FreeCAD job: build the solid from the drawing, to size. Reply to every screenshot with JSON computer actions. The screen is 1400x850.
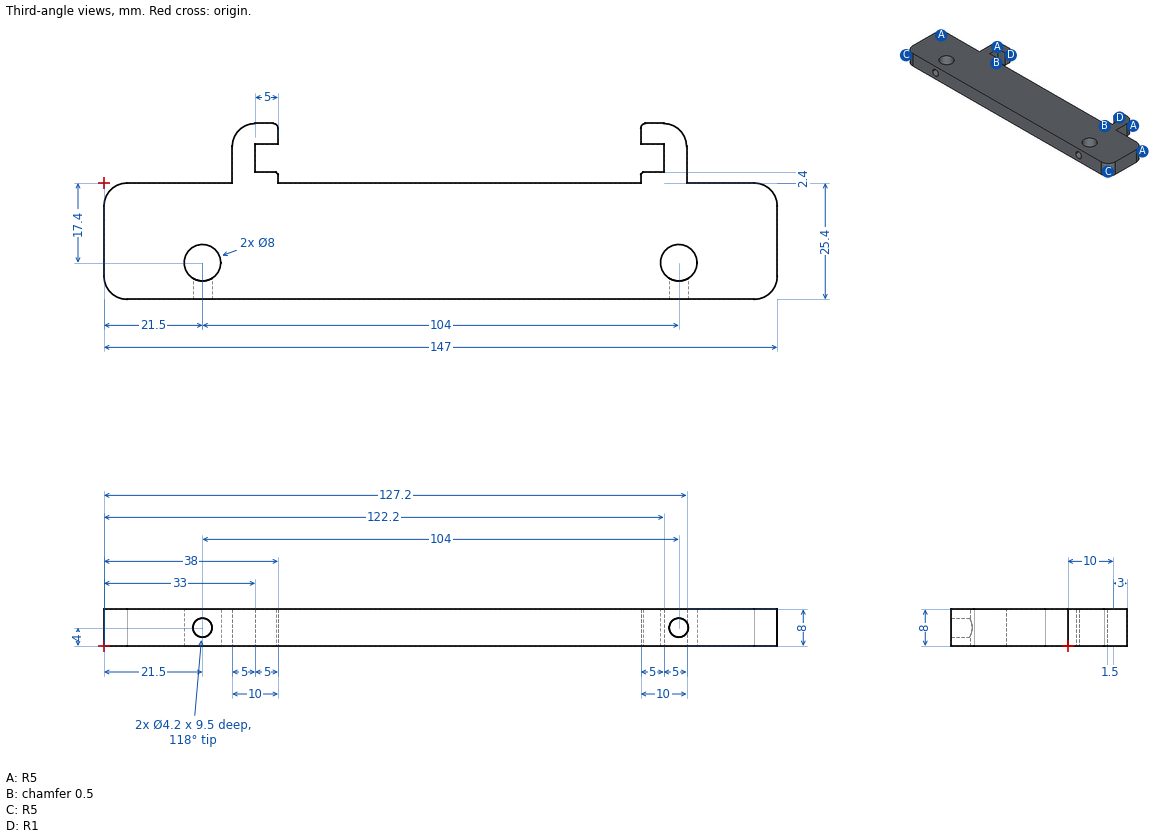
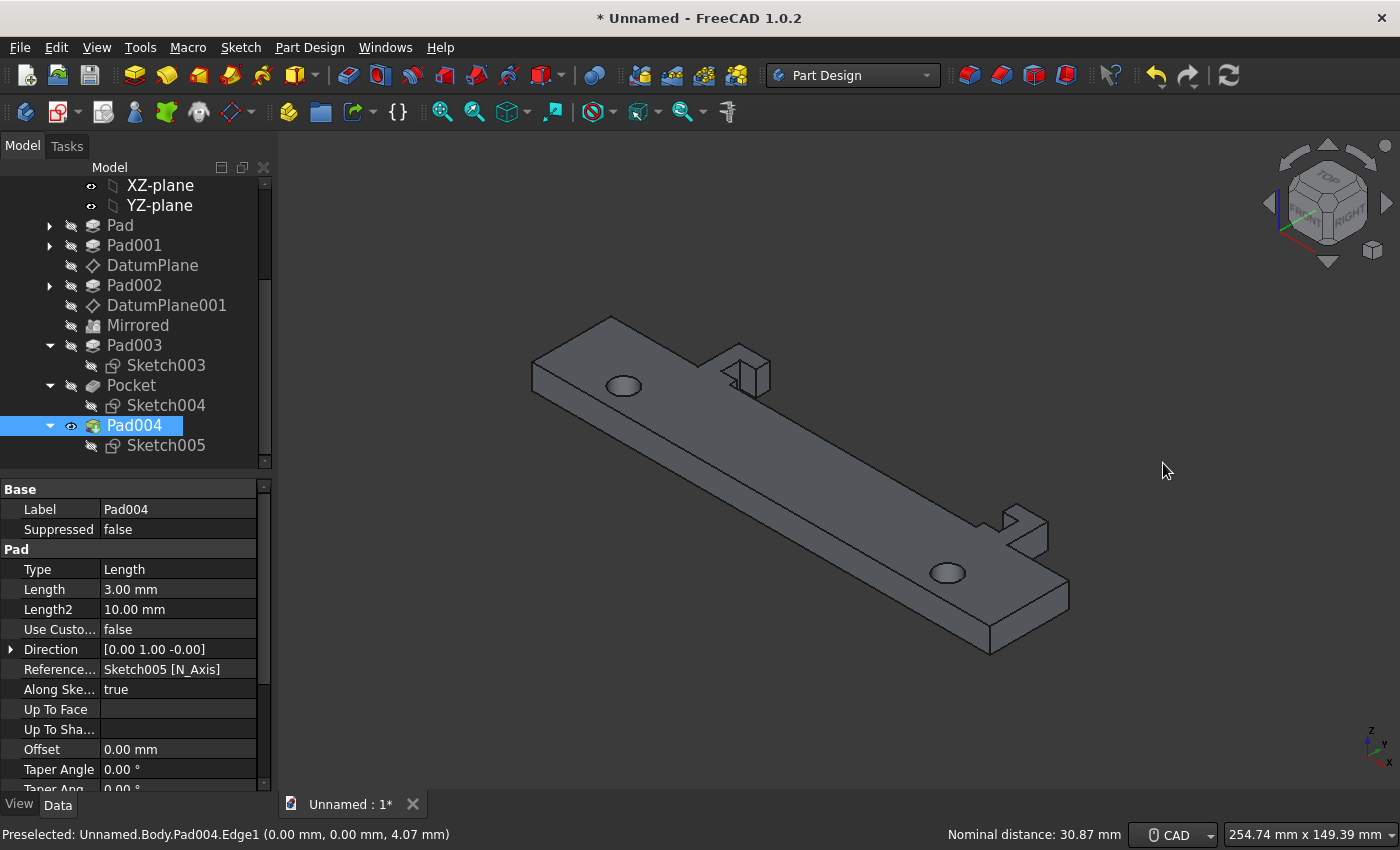
{"action": "key", "text": "2"}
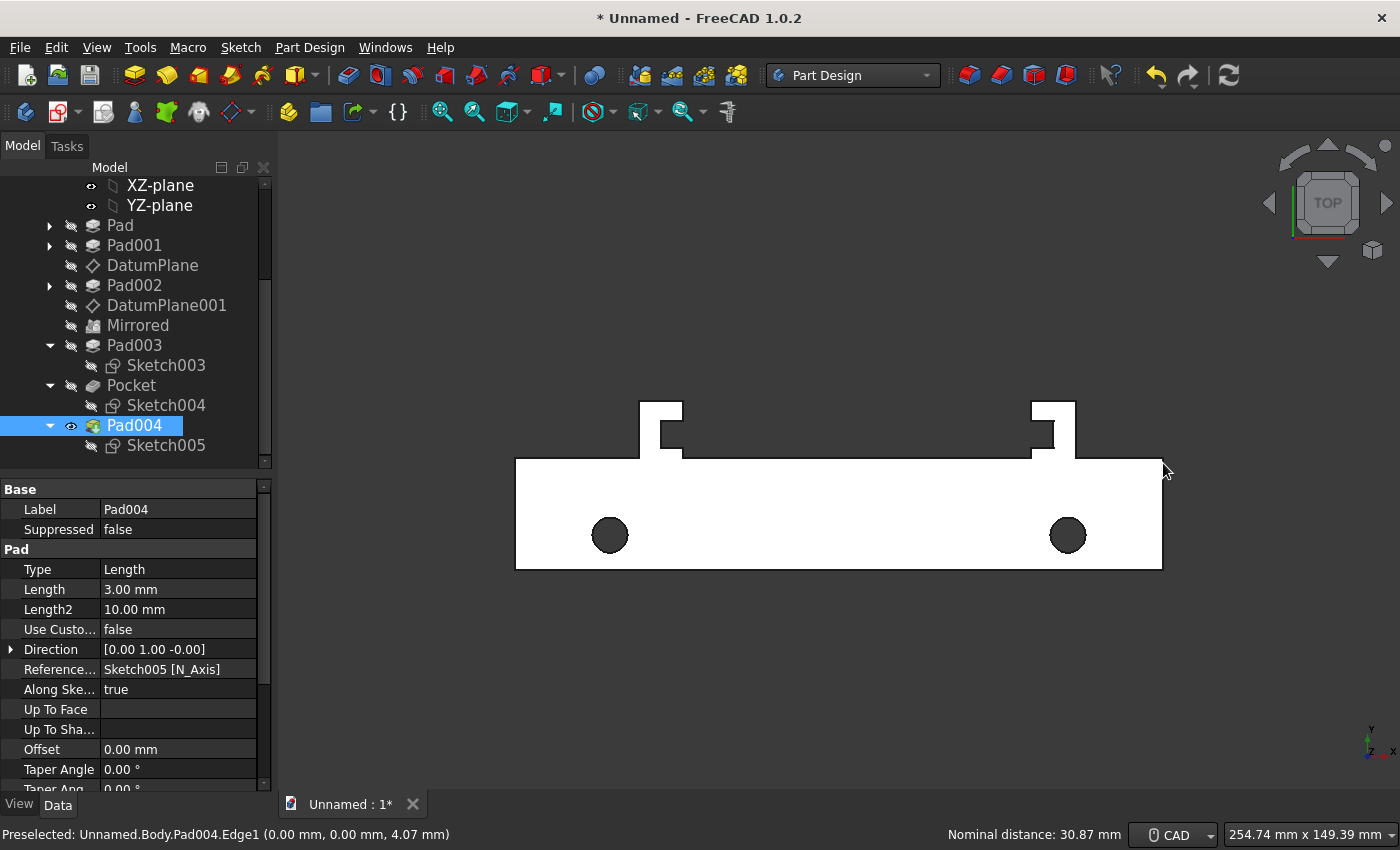
{"action": "key", "text": "1"}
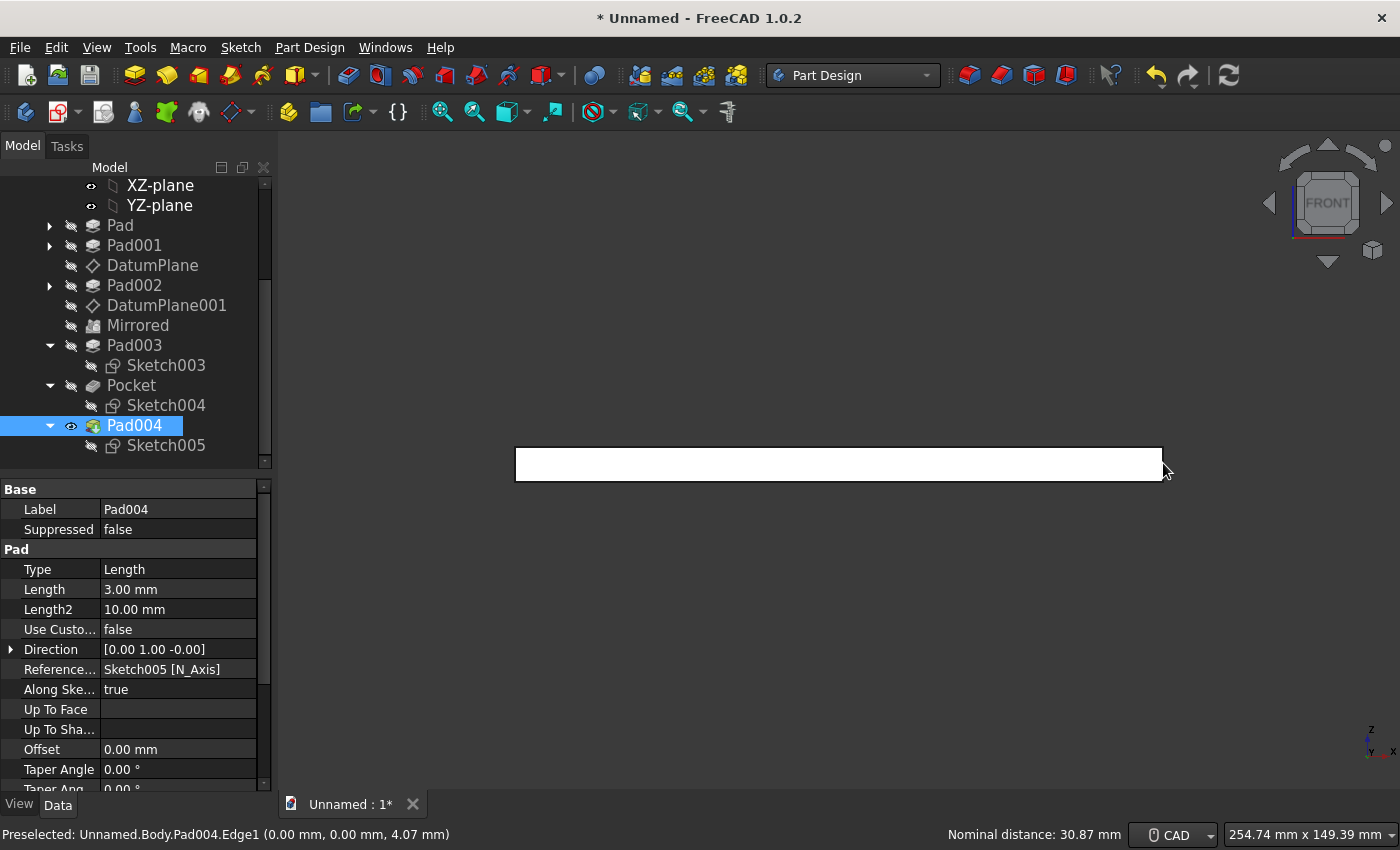
{"action": "key", "text": "3"}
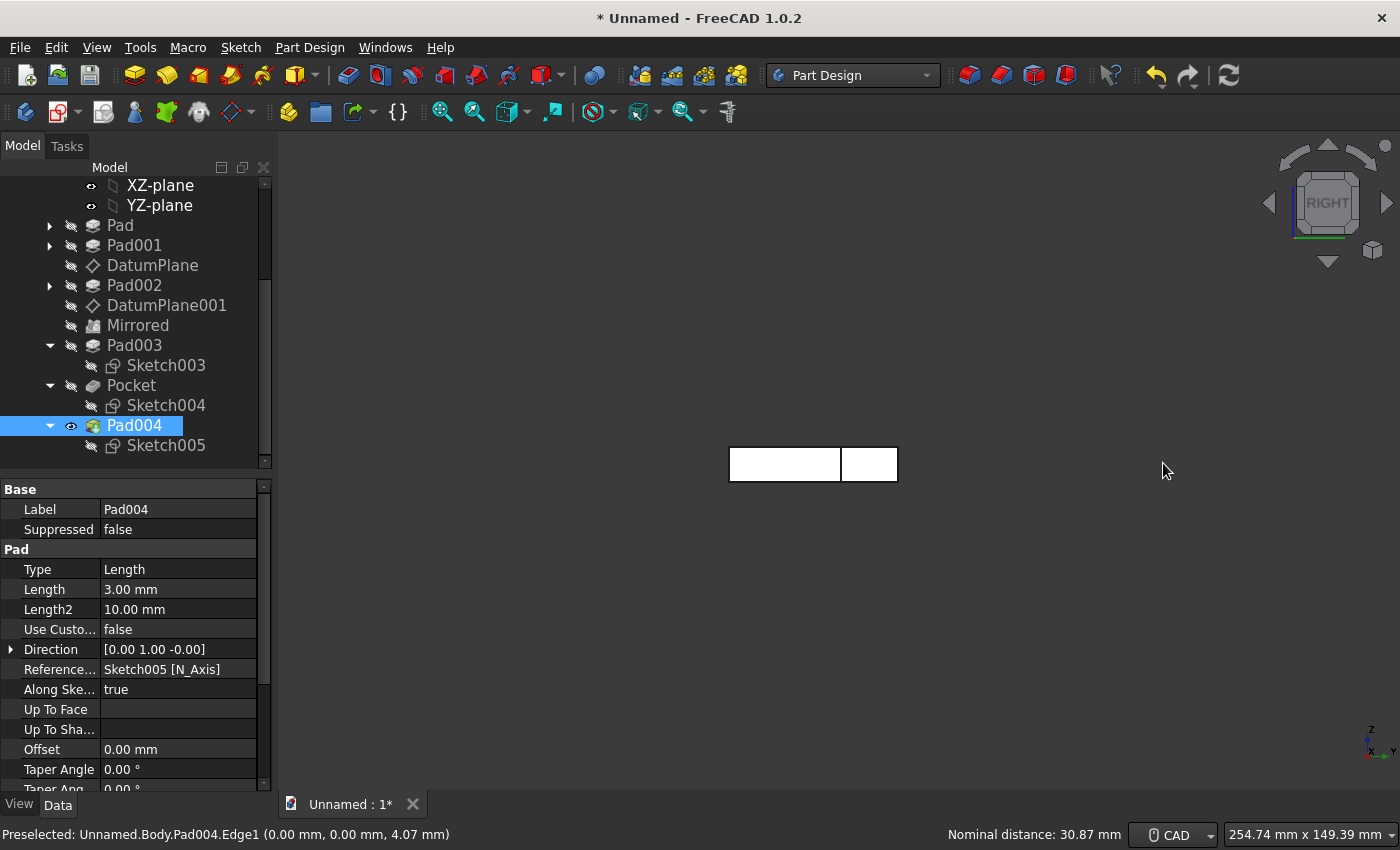
{"action": "left_click", "coordinate": [444, 112]}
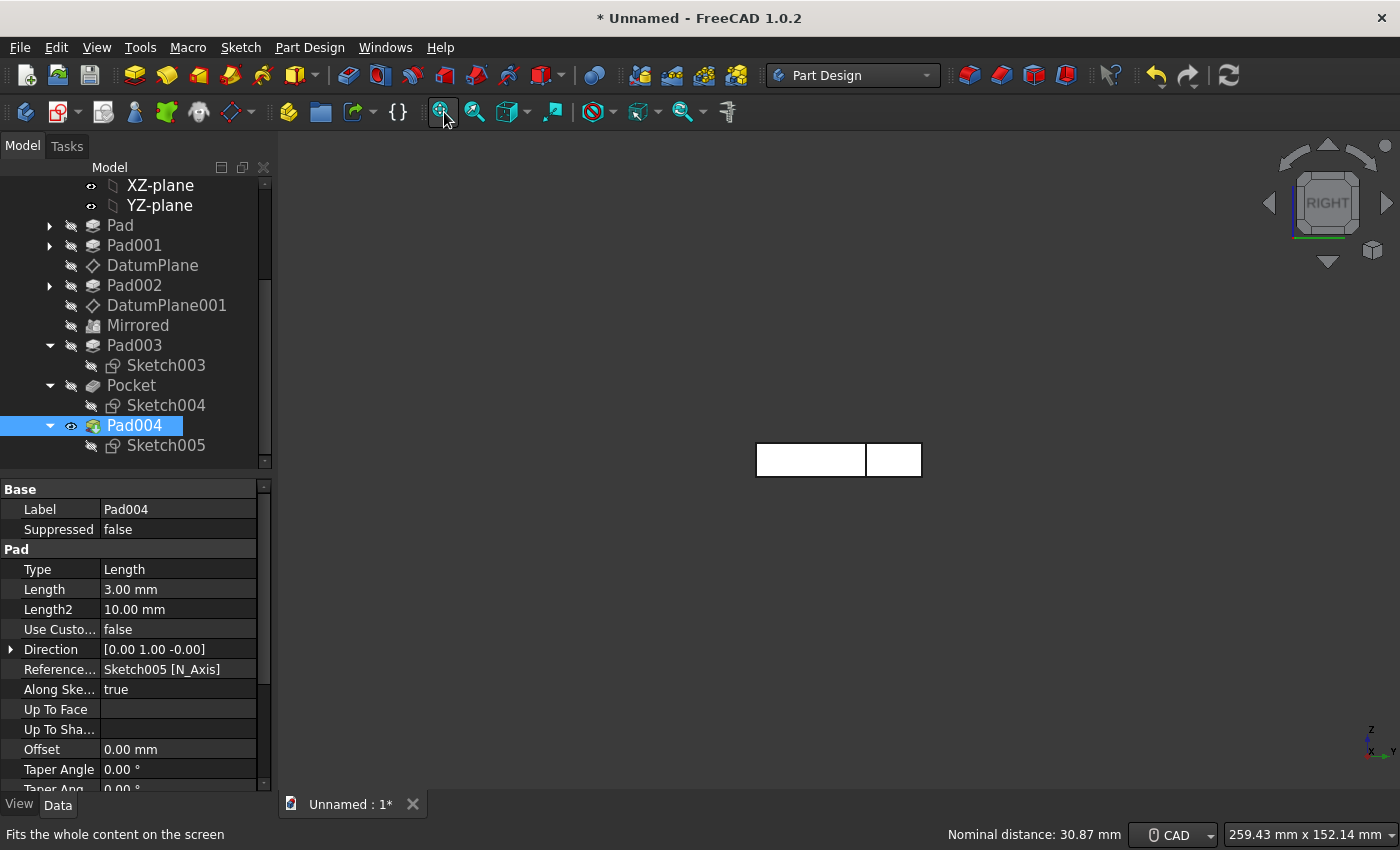
{"action": "left_click", "coordinate": [922, 459], "text": "ctrl"}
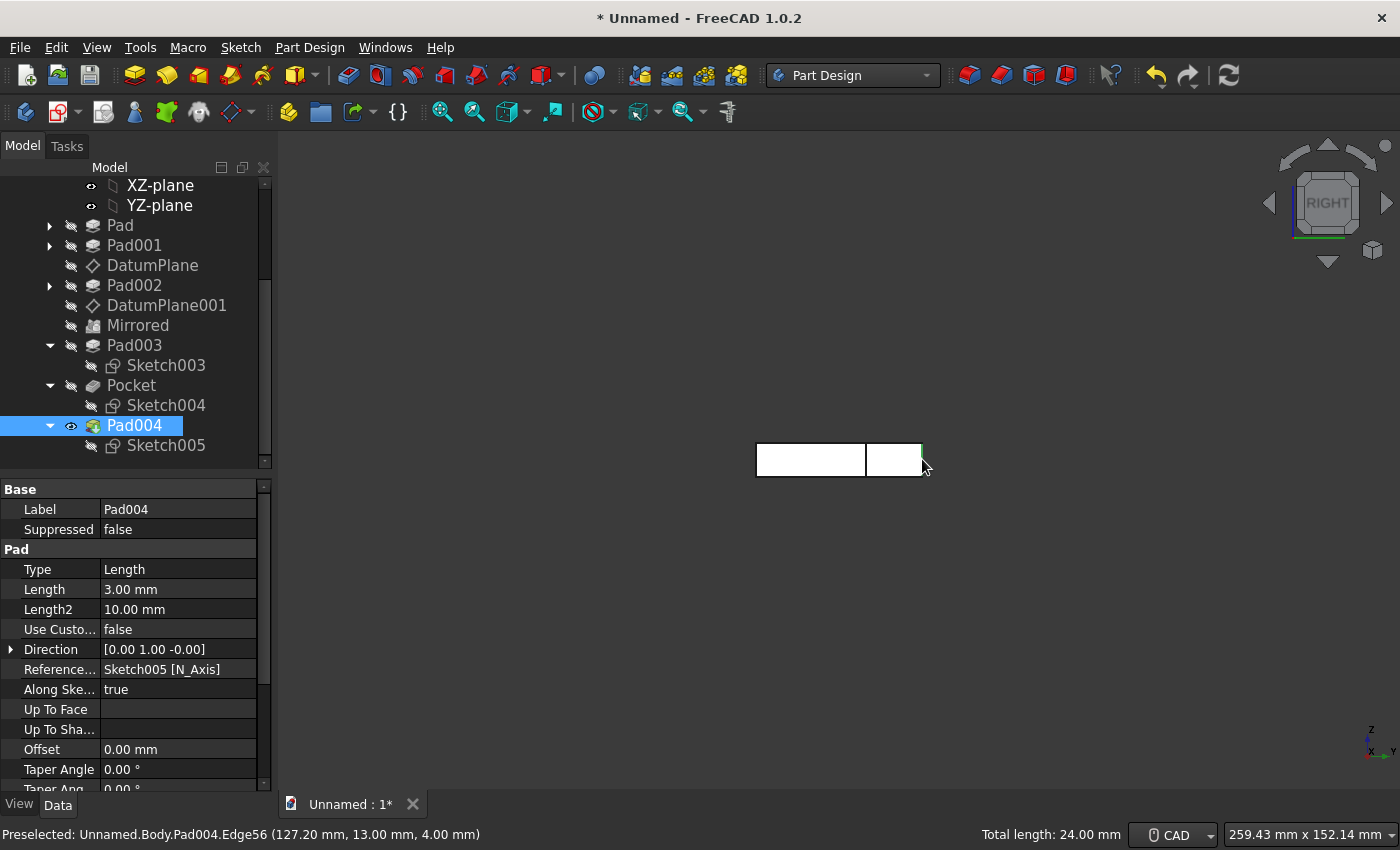
{"action": "left_click", "coordinate": [866, 459], "text": "ctrl"}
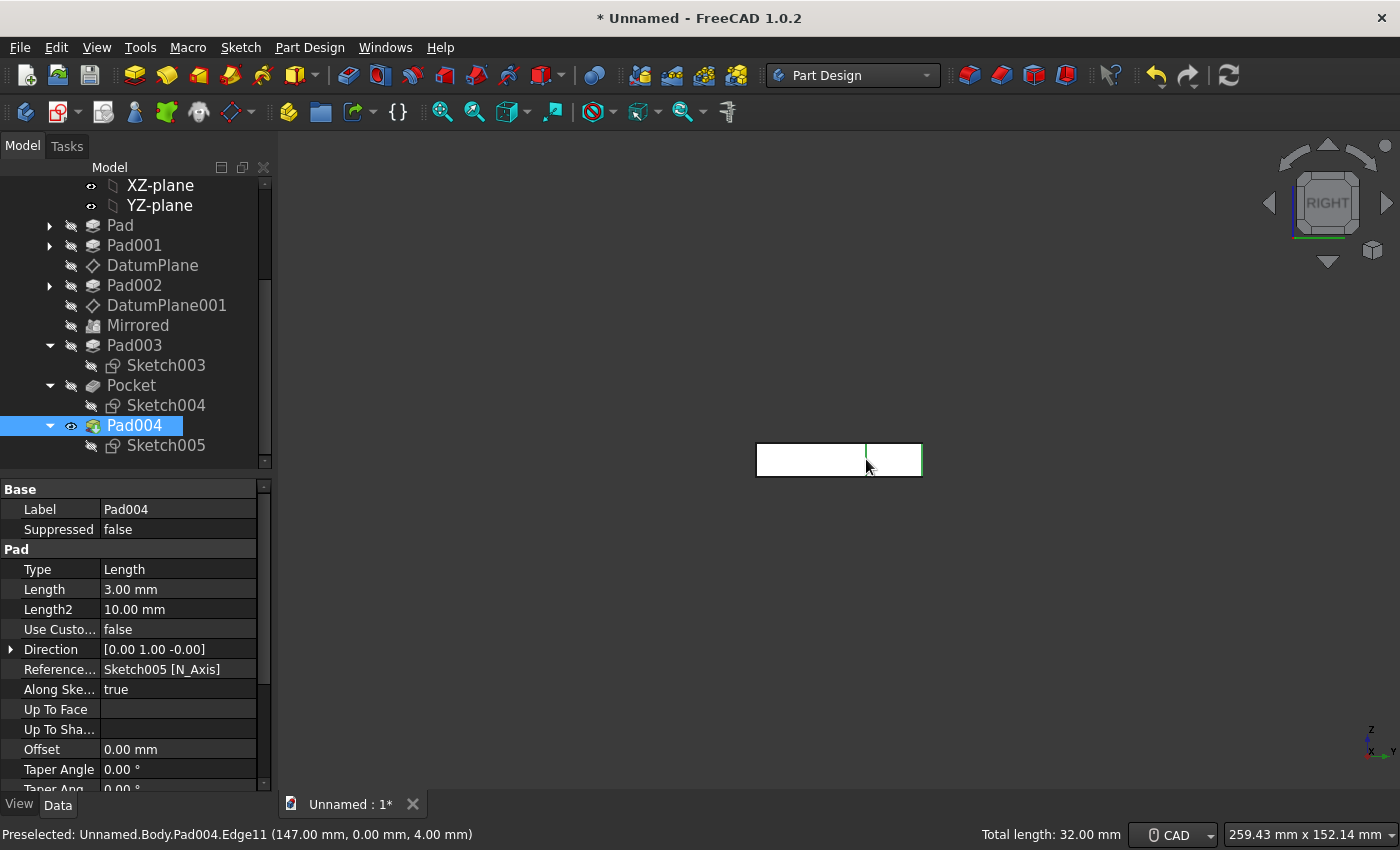
{"action": "left_click", "coordinate": [970, 76]}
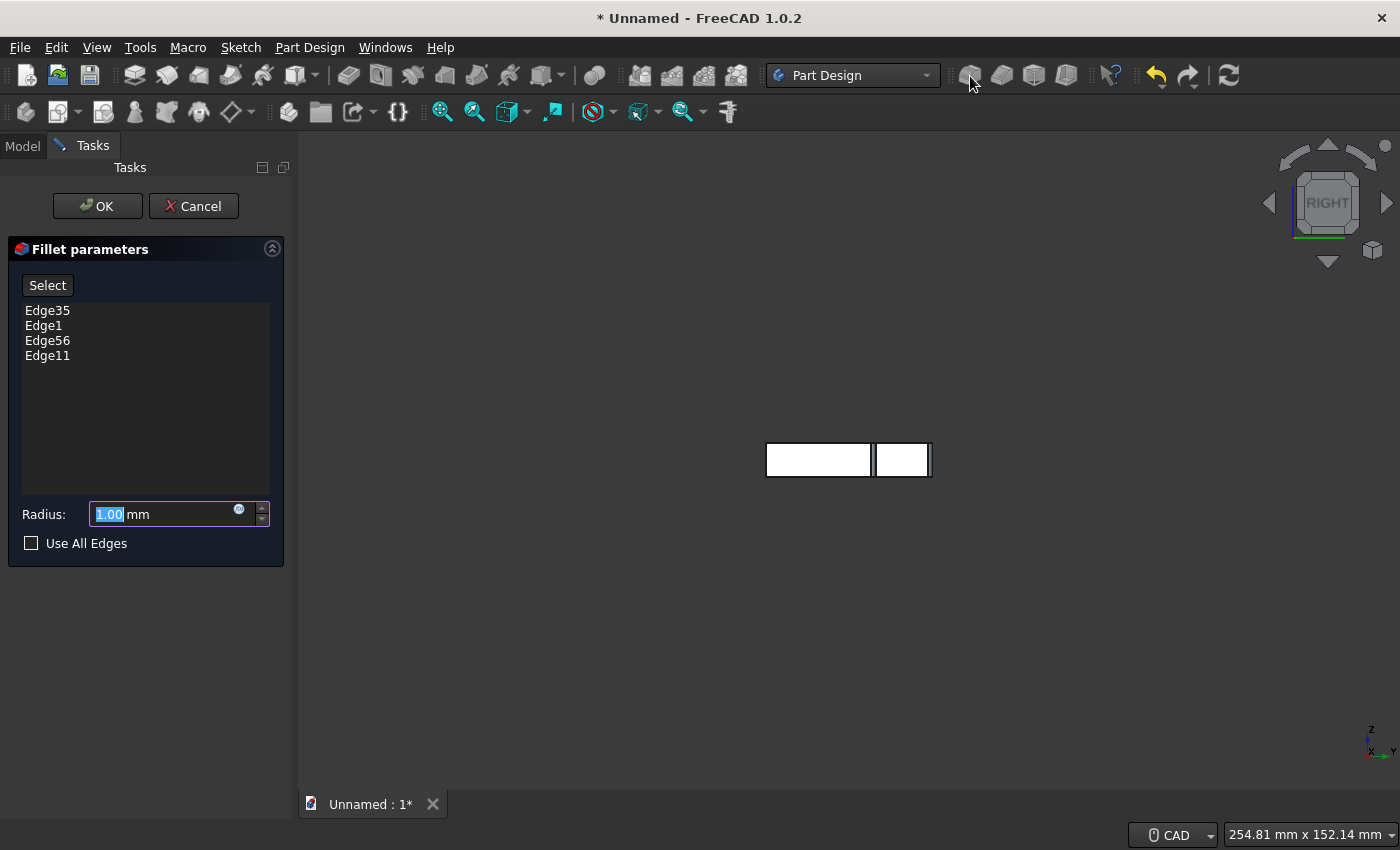
{"action": "type", "text": "5"}
{"action": "key", "text": "Tab"}